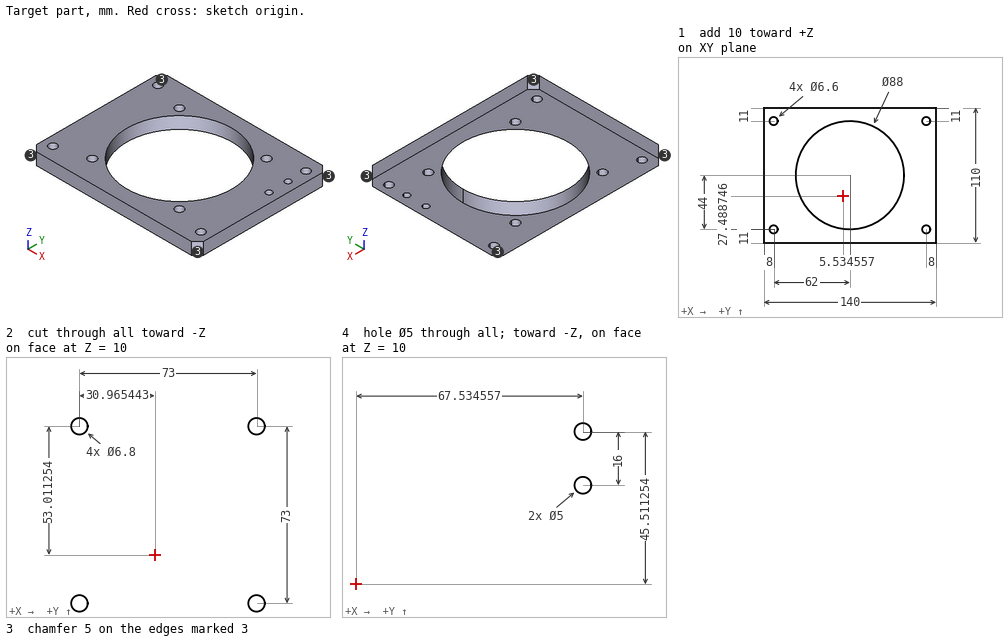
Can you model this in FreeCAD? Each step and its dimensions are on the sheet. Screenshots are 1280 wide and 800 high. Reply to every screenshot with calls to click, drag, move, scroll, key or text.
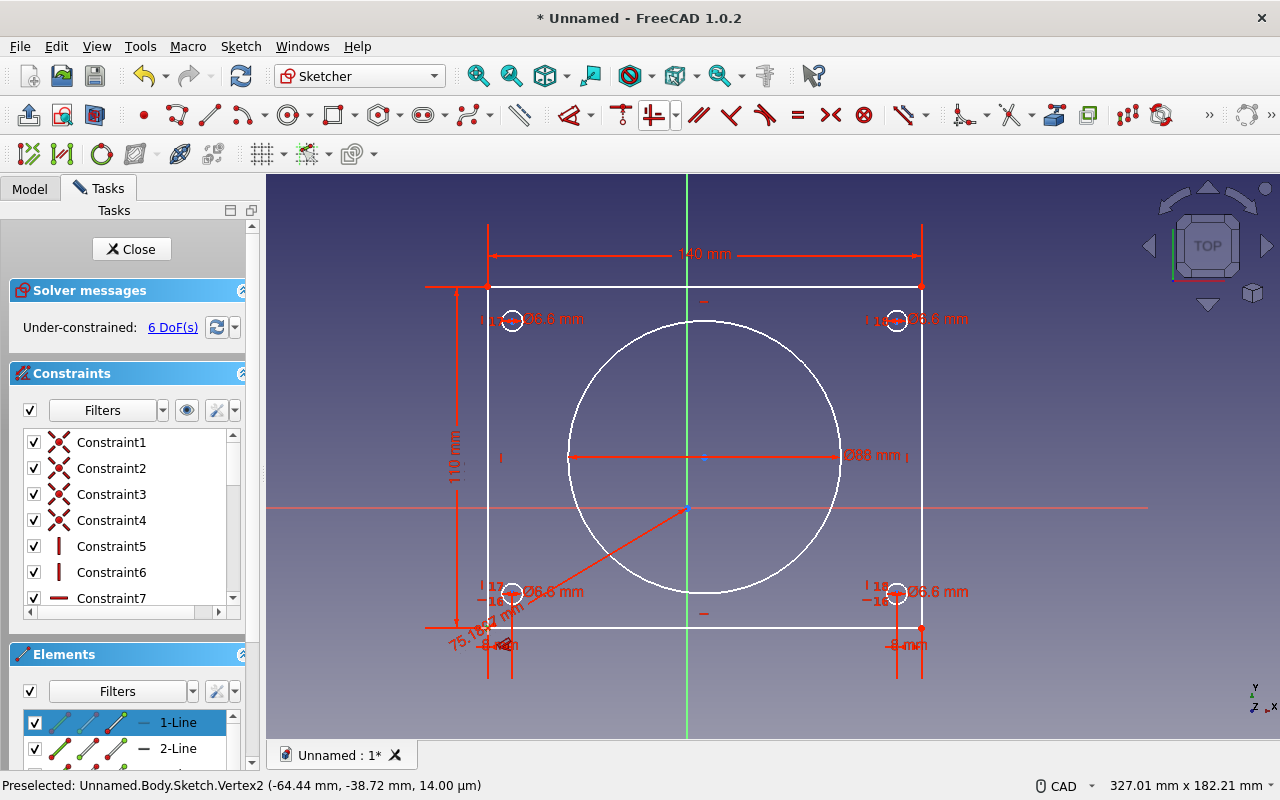
click(512, 594)
click(454, 611)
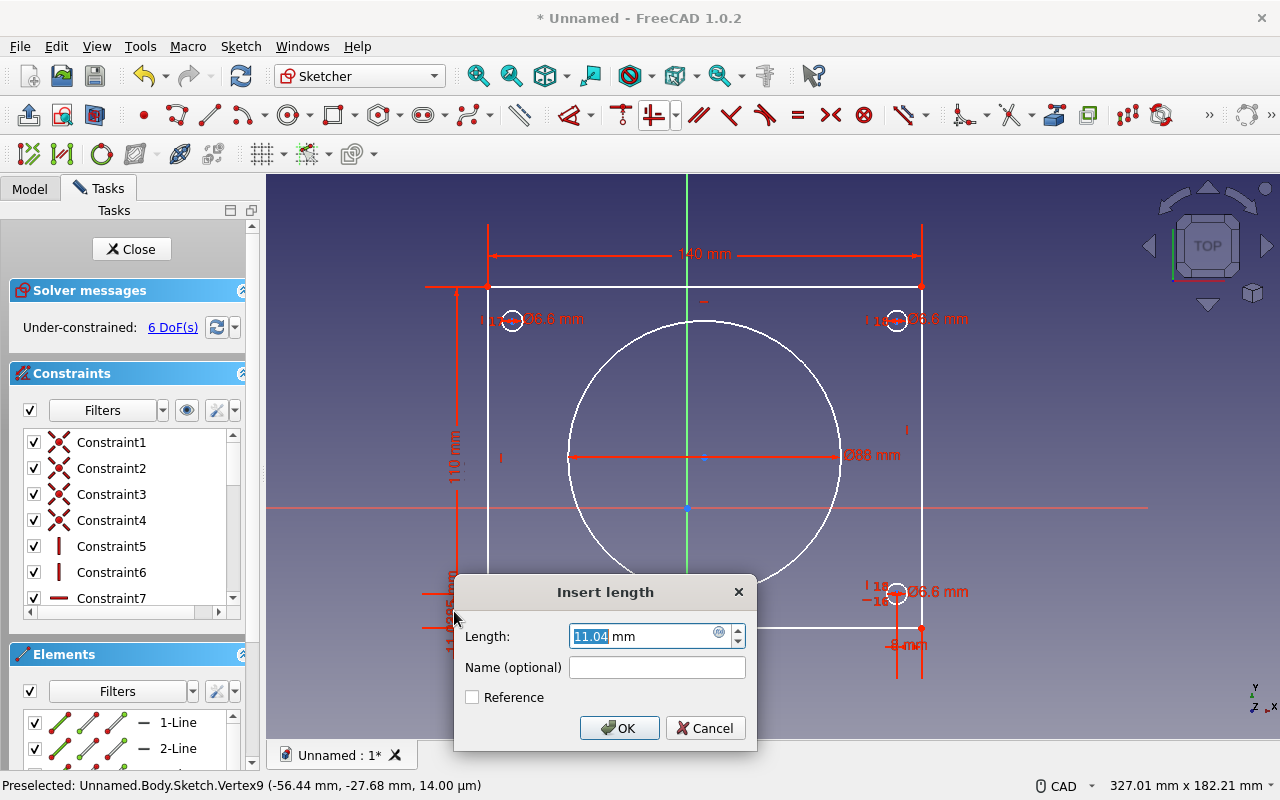
text(11)
key(Return)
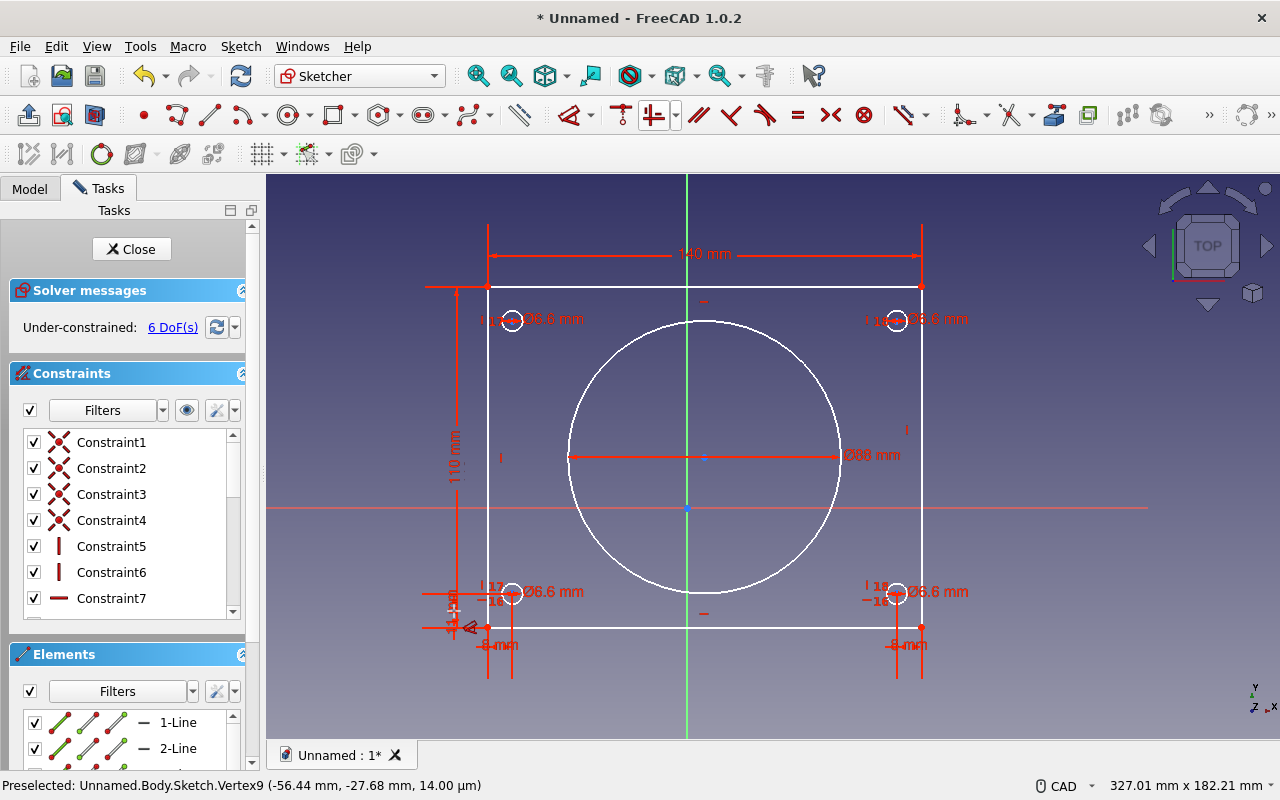
click(512, 594)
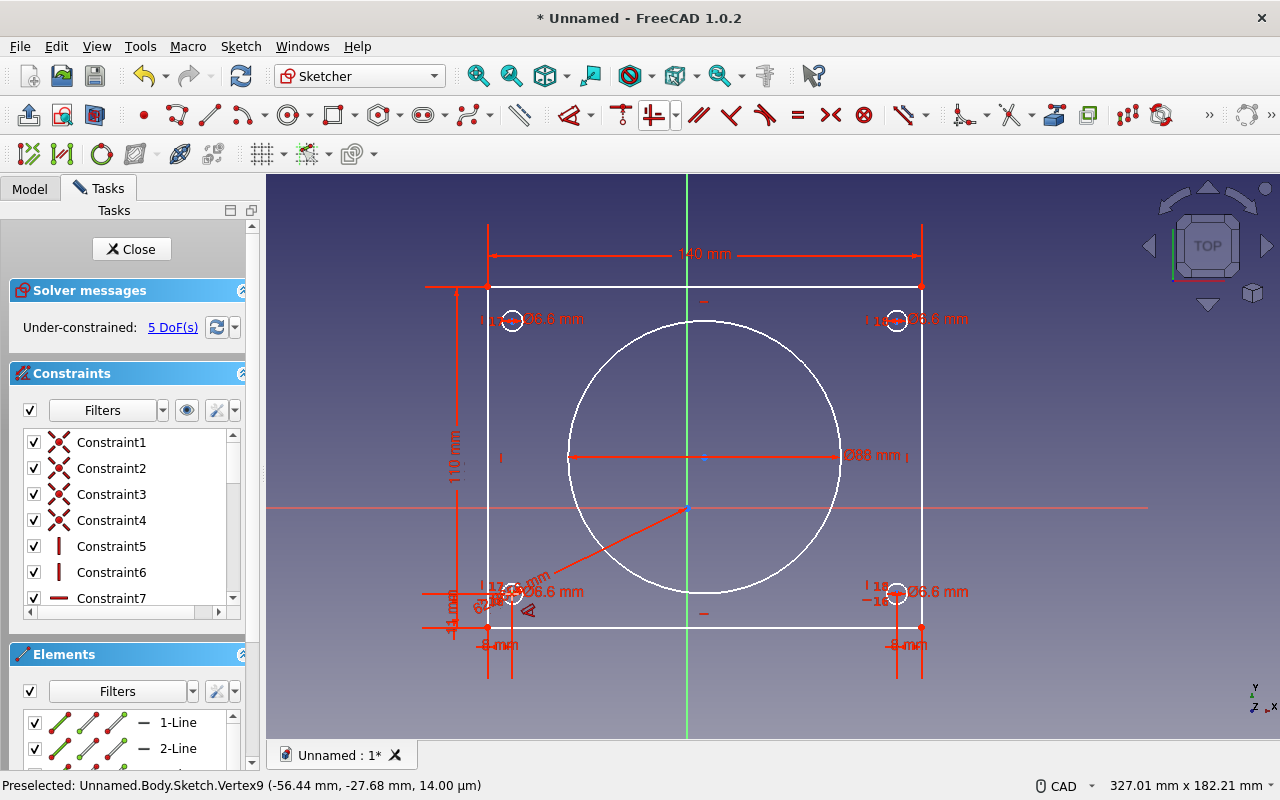
click(705, 457)
click(608, 423)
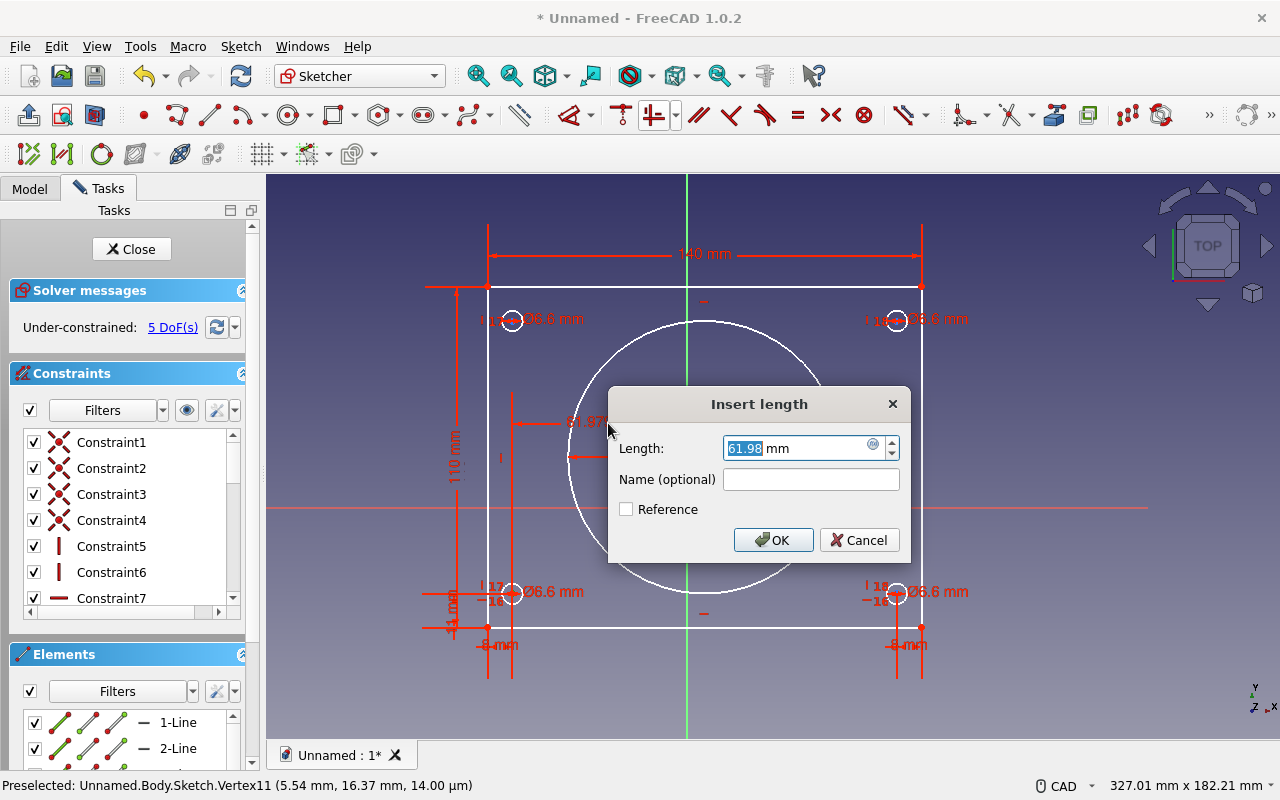
text(62)
key(Return)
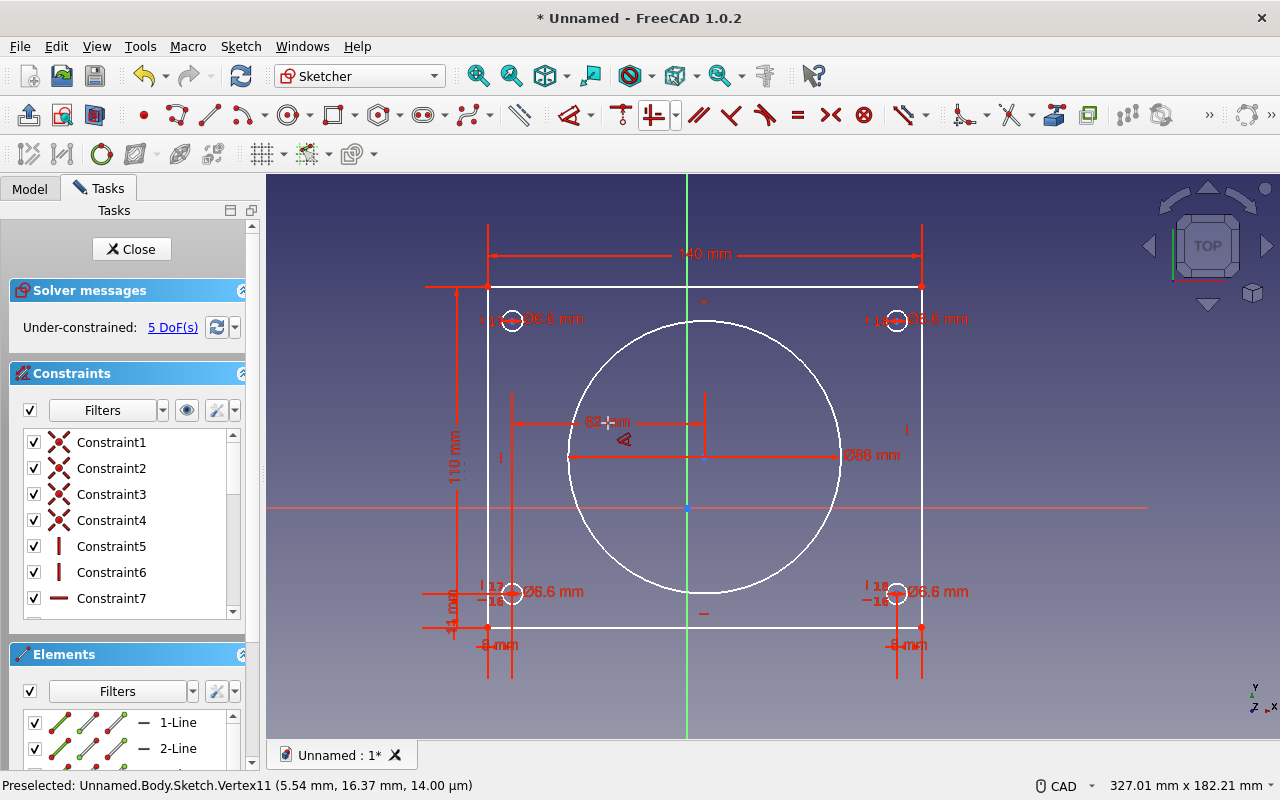
click(512, 594)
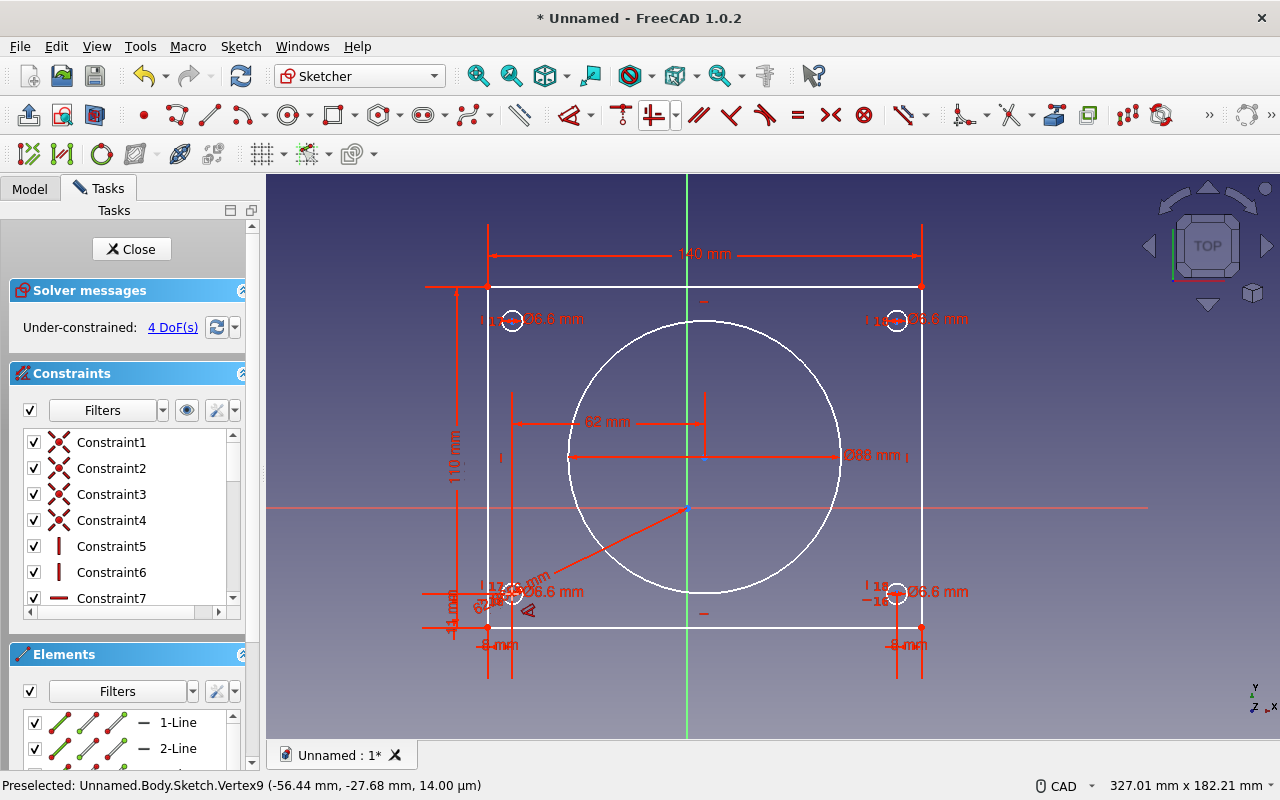
click(705, 457)
click(739, 526)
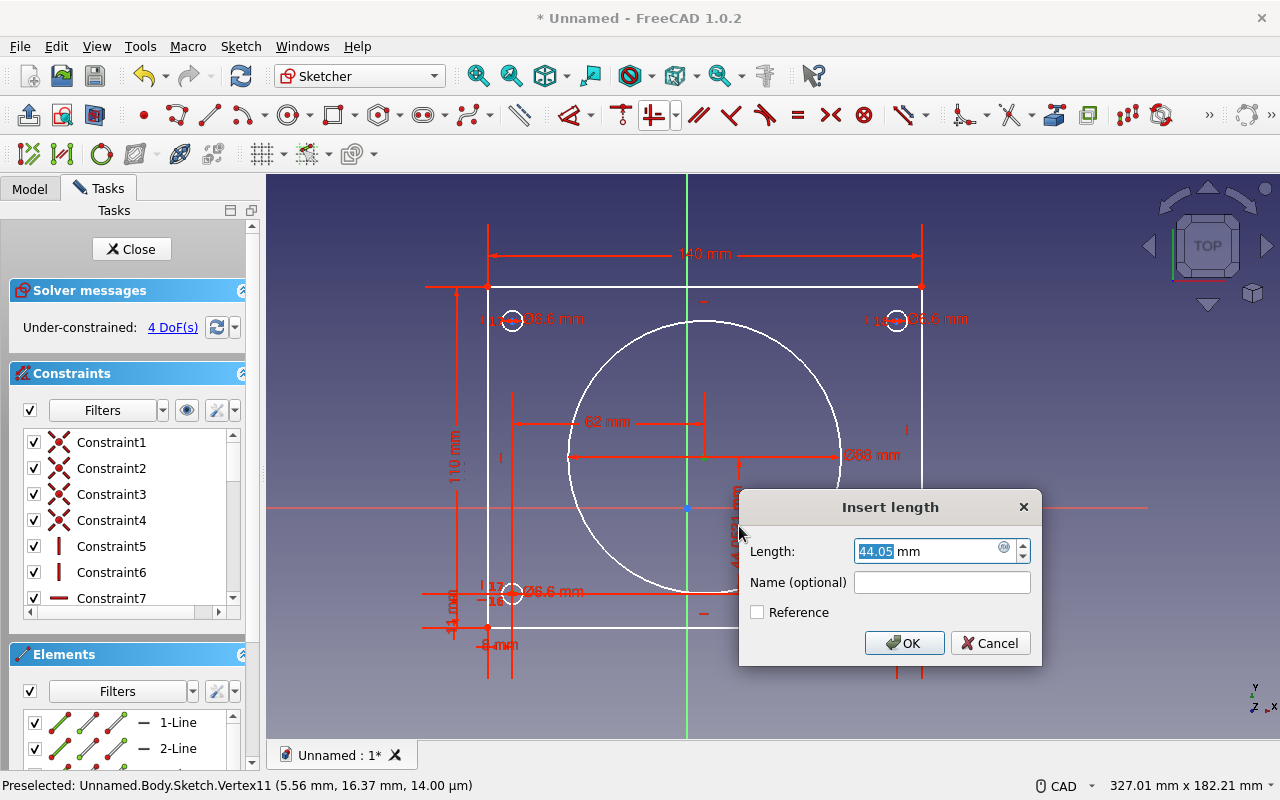
text(44)
key(Return)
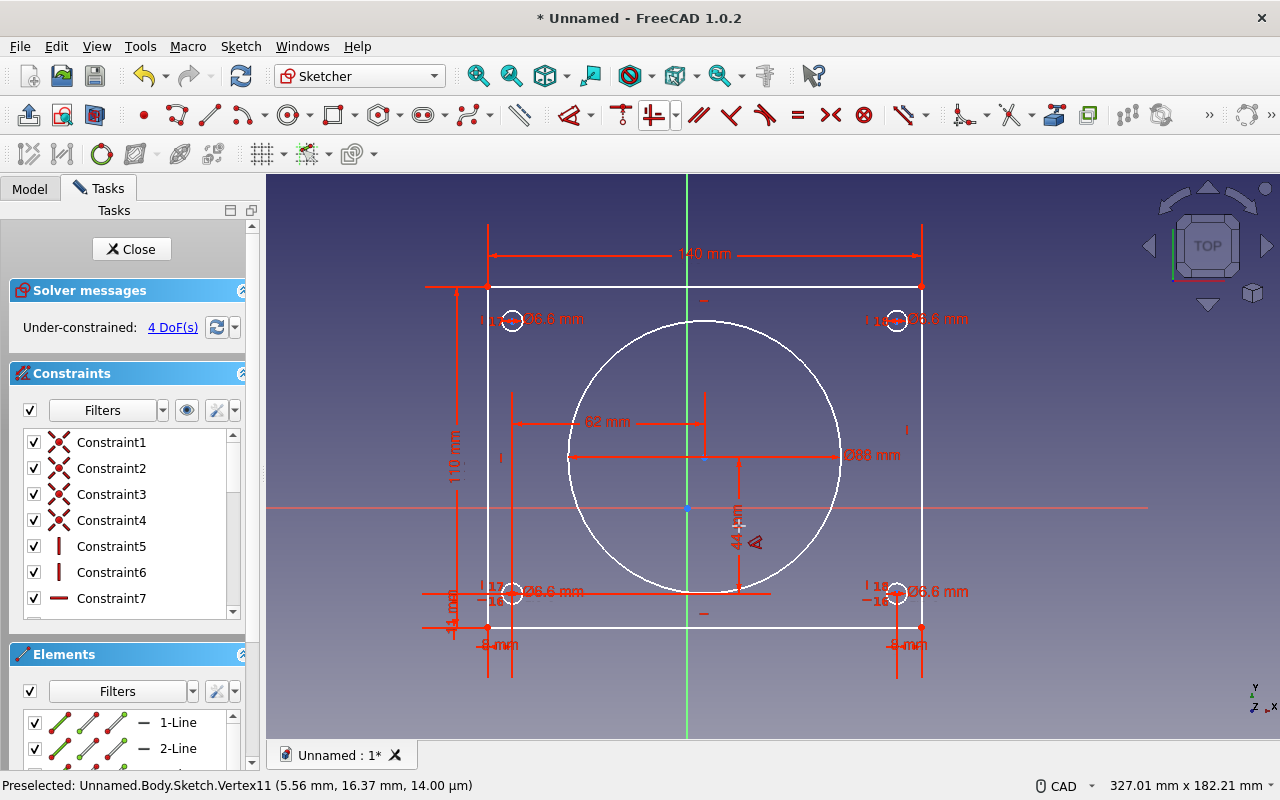
click(488, 287)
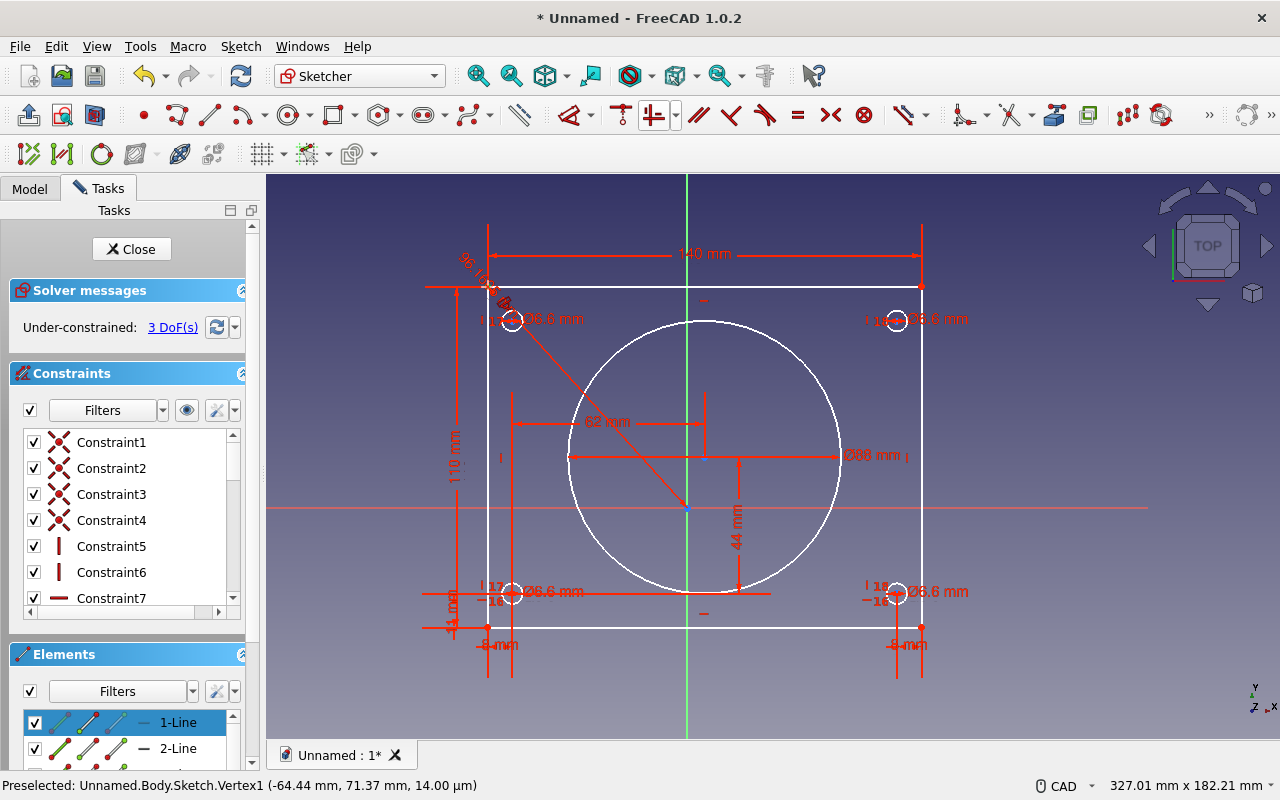
click(512, 321)
click(454, 304)